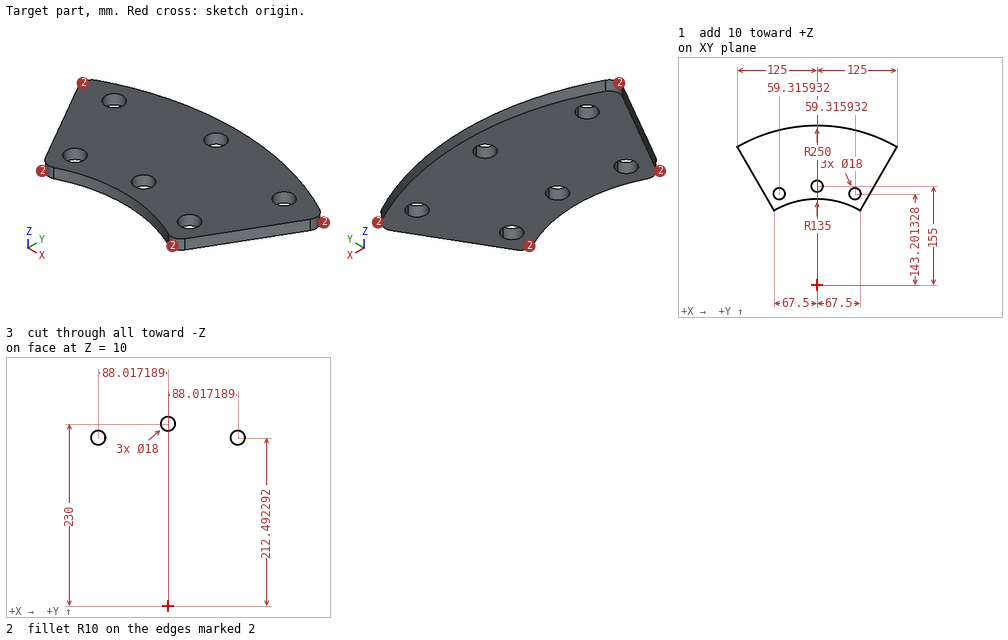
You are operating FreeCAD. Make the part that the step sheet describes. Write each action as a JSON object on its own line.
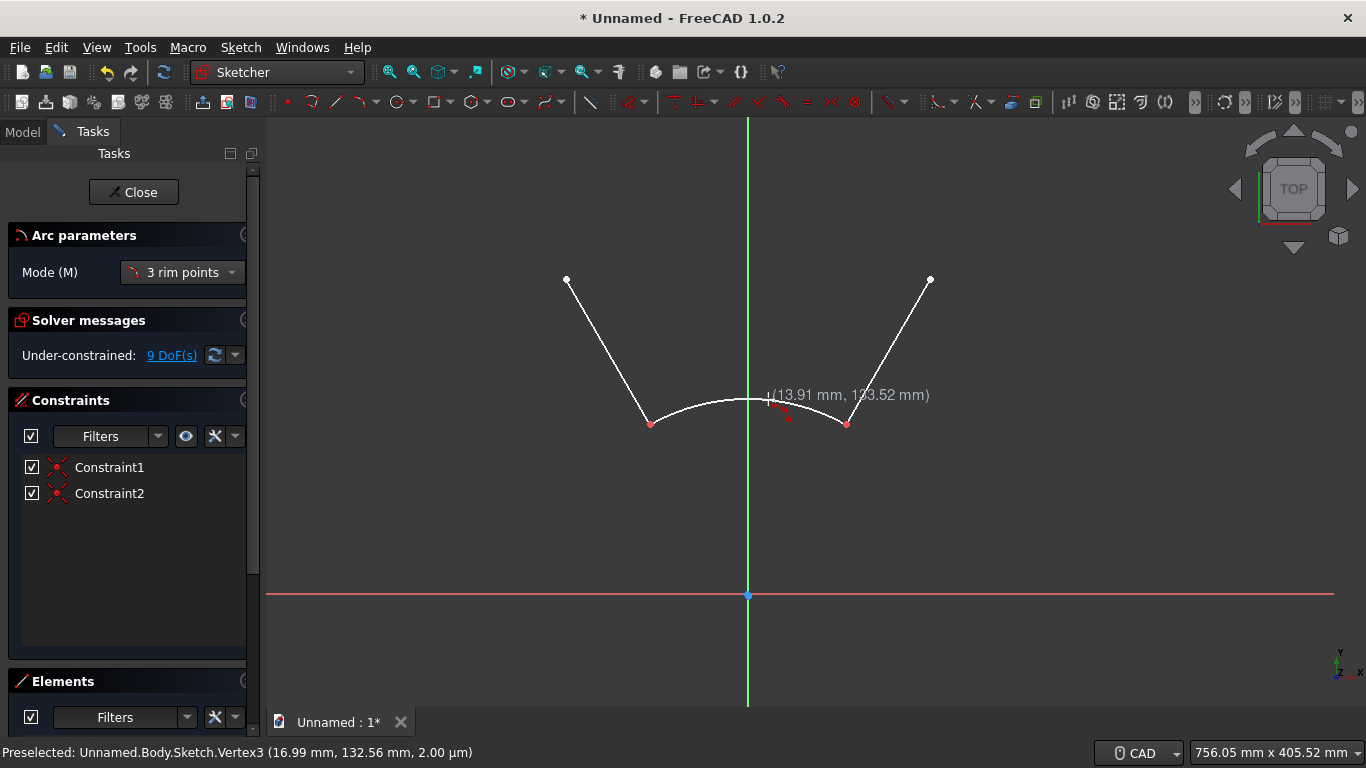
{"action": "left_click", "coordinate": [930, 280]}
{"action": "left_click", "coordinate": [566, 280]}
{"action": "left_click", "coordinate": [786, 233]}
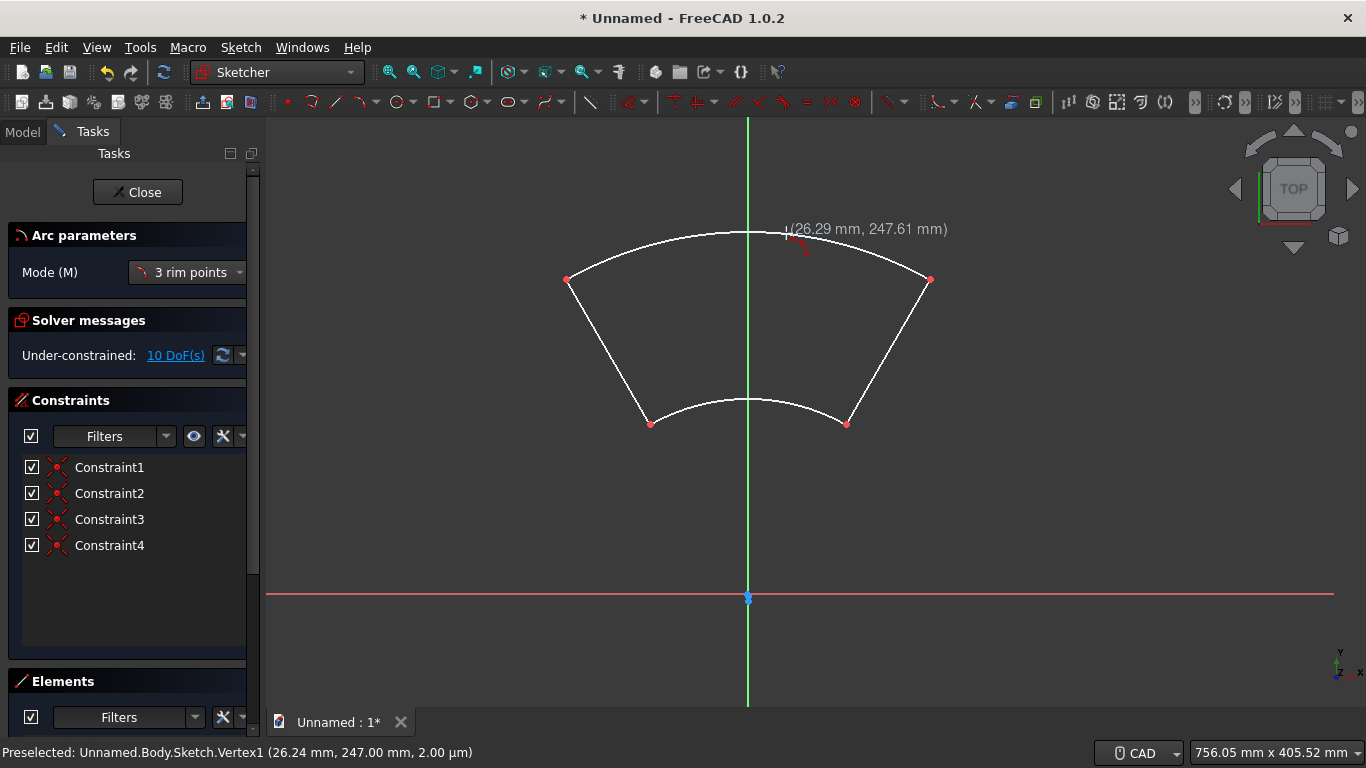
{"action": "left_click", "coordinate": [398, 102]}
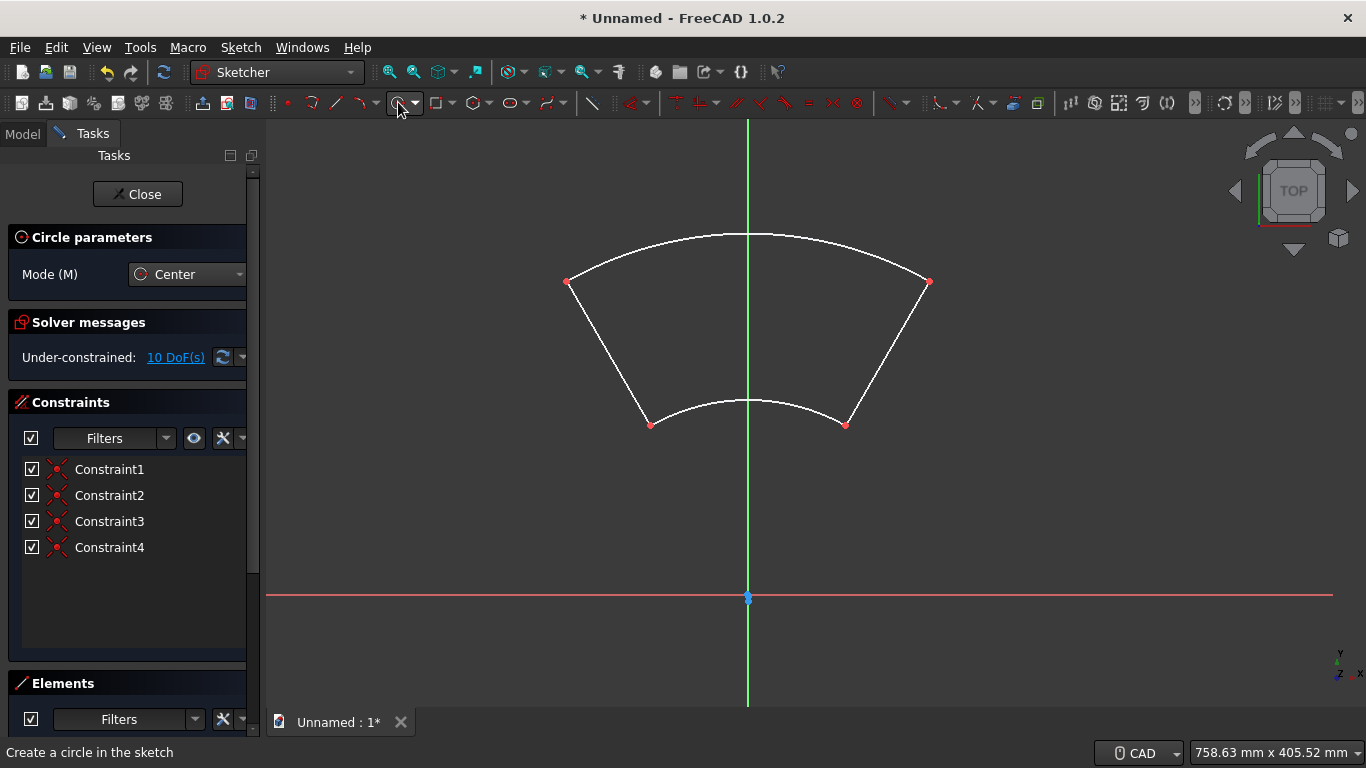
{"action": "scroll", "coordinate": [834, 387], "scroll_direction": "up", "scroll_amount": 3}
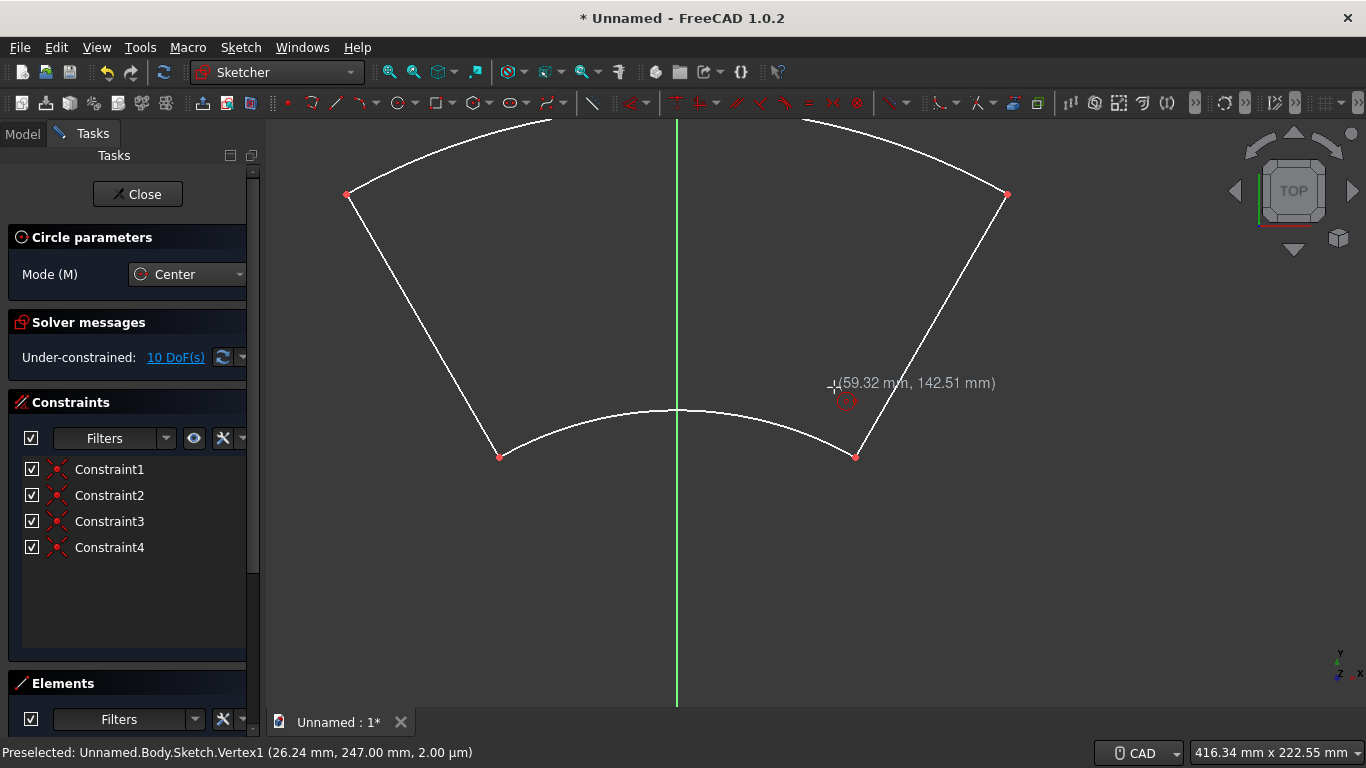
{"action": "left_click", "coordinate": [834, 387]}
{"action": "mouse_move", "coordinate": [850, 370]}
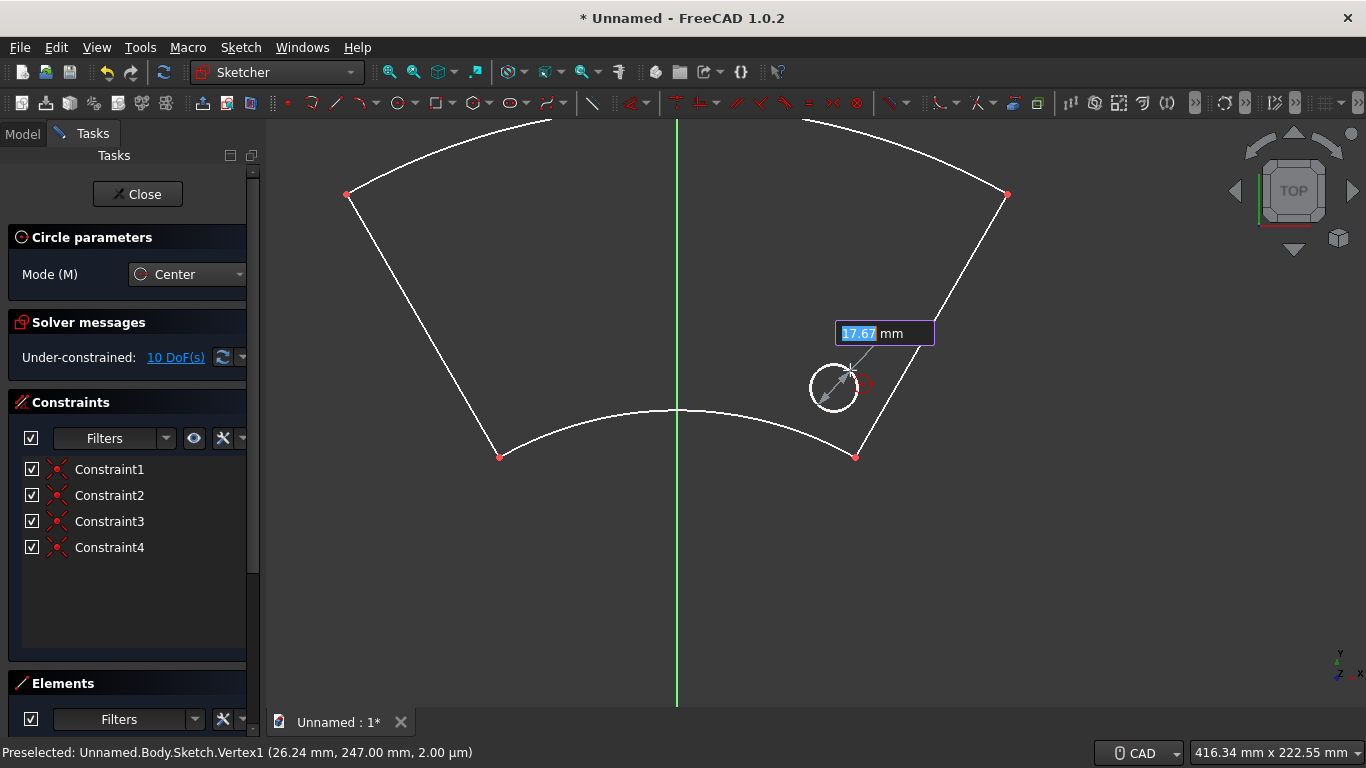
{"action": "type", "text": "18"}
{"action": "key", "text": "Return"}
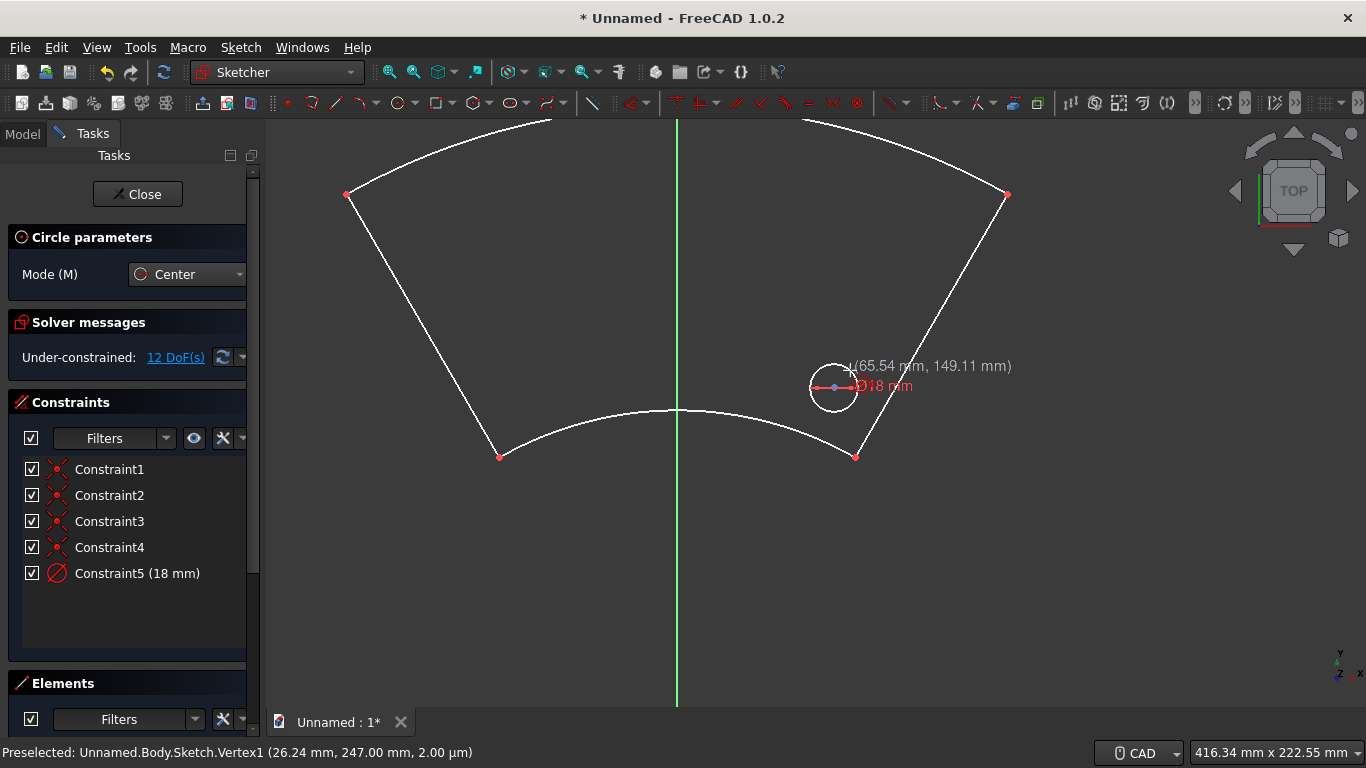
{"action": "left_click", "coordinate": [520, 387]}
{"action": "mouse_move", "coordinate": [537, 370]}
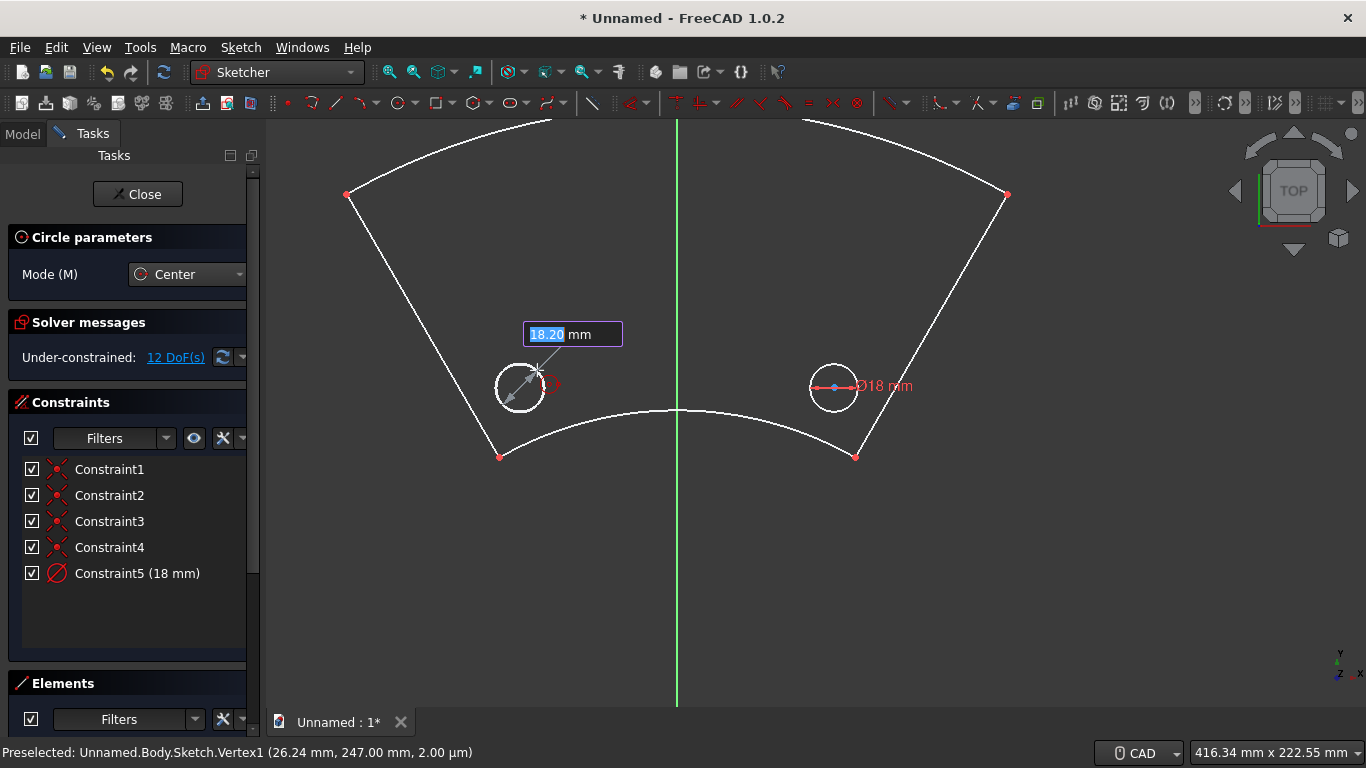
{"action": "type", "text": "18"}
{"action": "key", "text": "Return"}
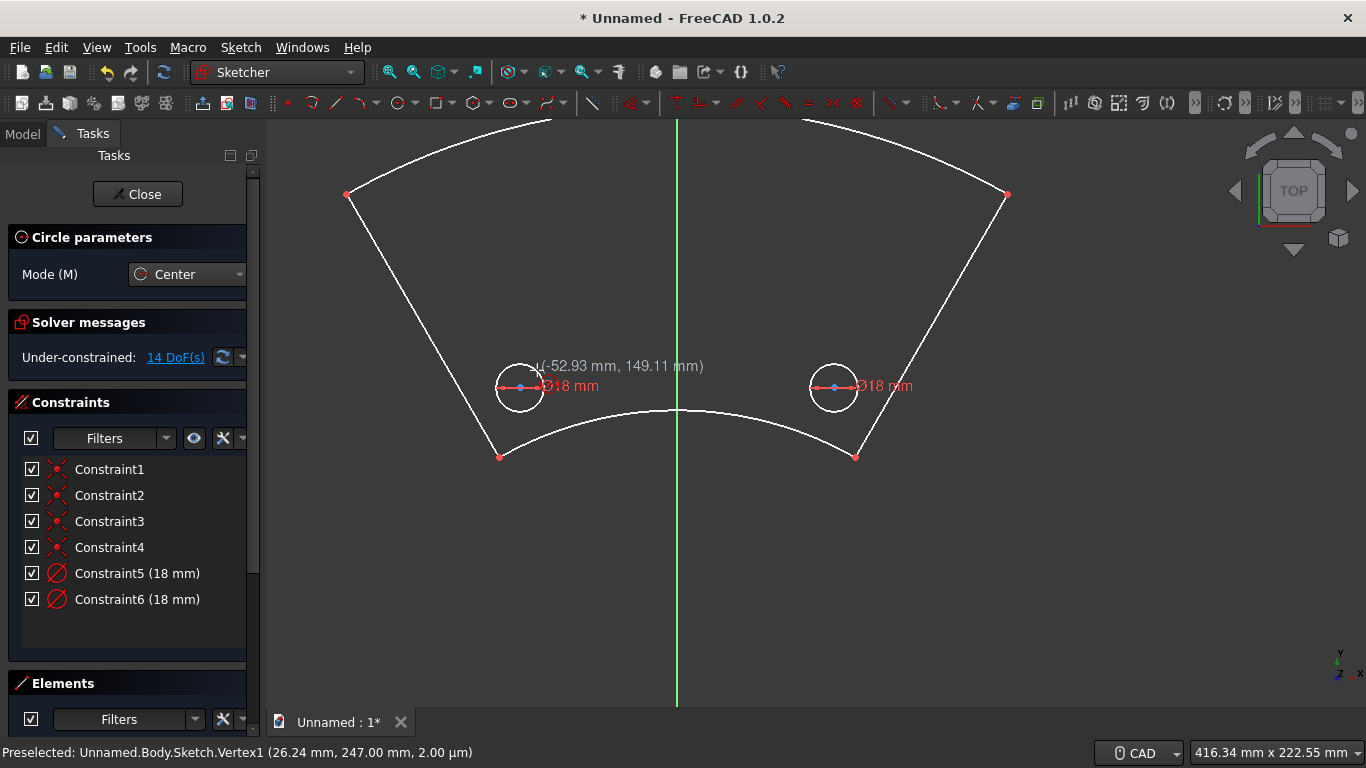
{"action": "left_click", "coordinate": [677, 355]}
{"action": "mouse_move", "coordinate": [694, 339]}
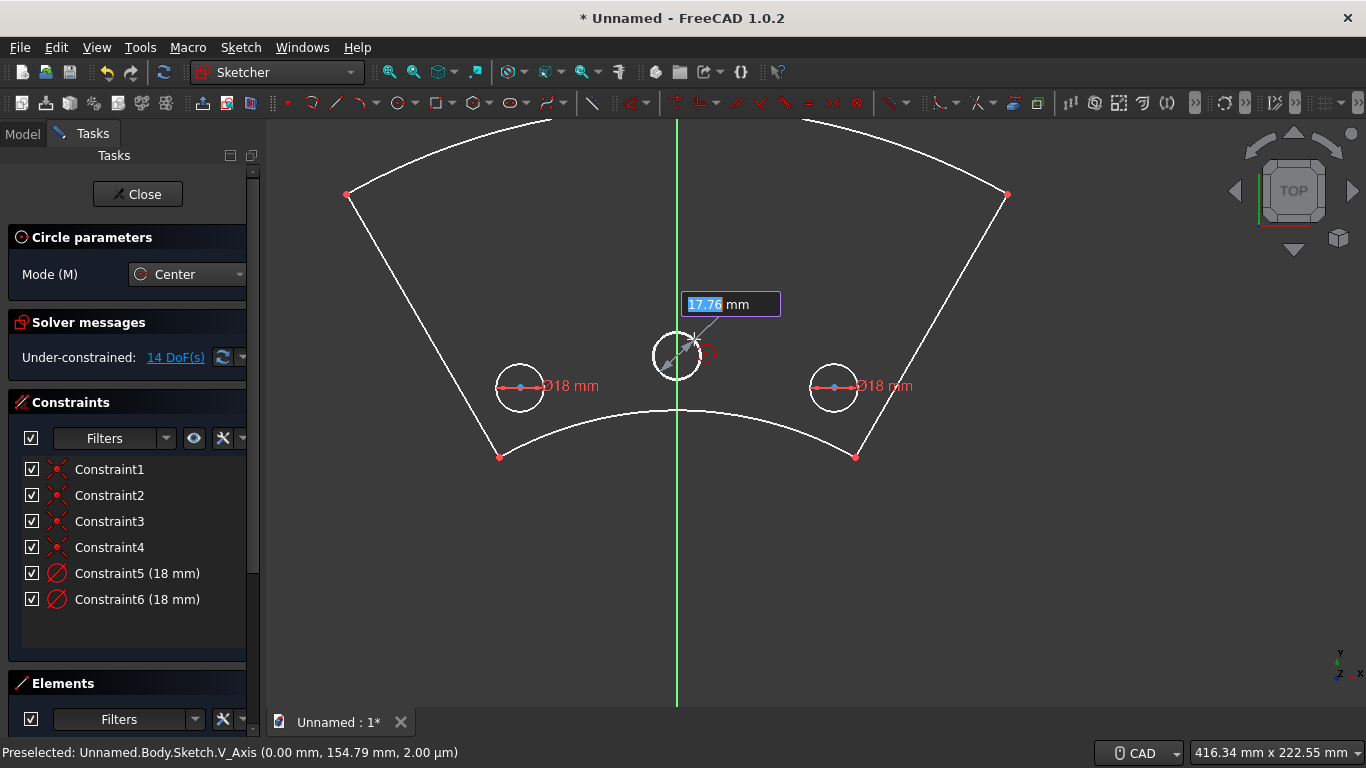
{"action": "type", "text": "18"}
{"action": "key", "text": "Return"}
{"action": "key", "text": "Escape"}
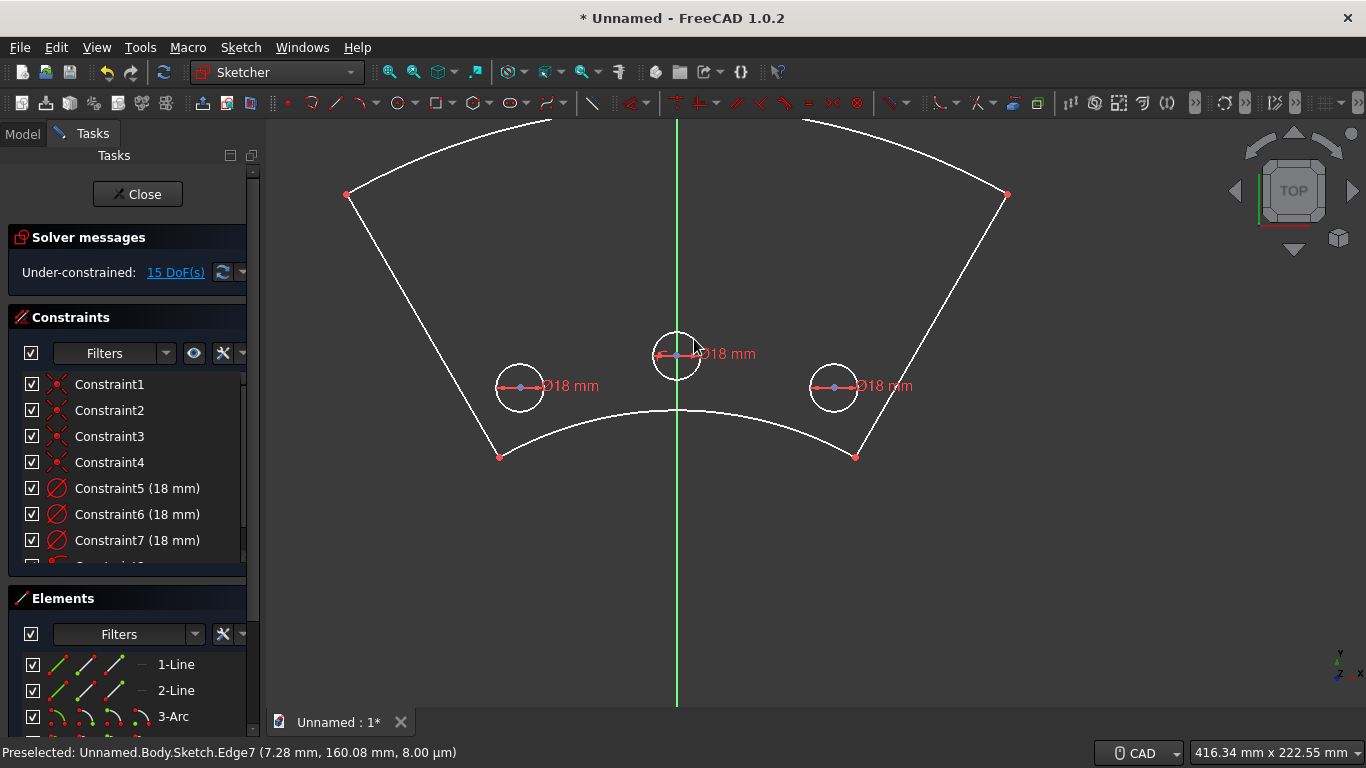
{"action": "left_click", "coordinate": [751, 418]}